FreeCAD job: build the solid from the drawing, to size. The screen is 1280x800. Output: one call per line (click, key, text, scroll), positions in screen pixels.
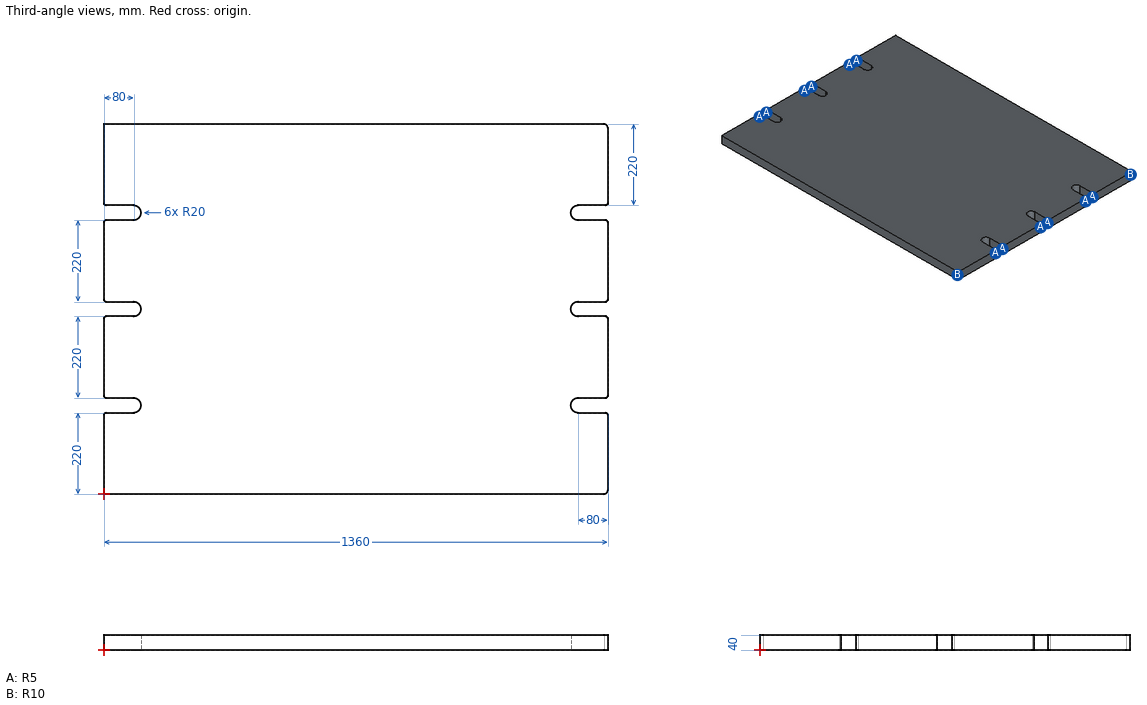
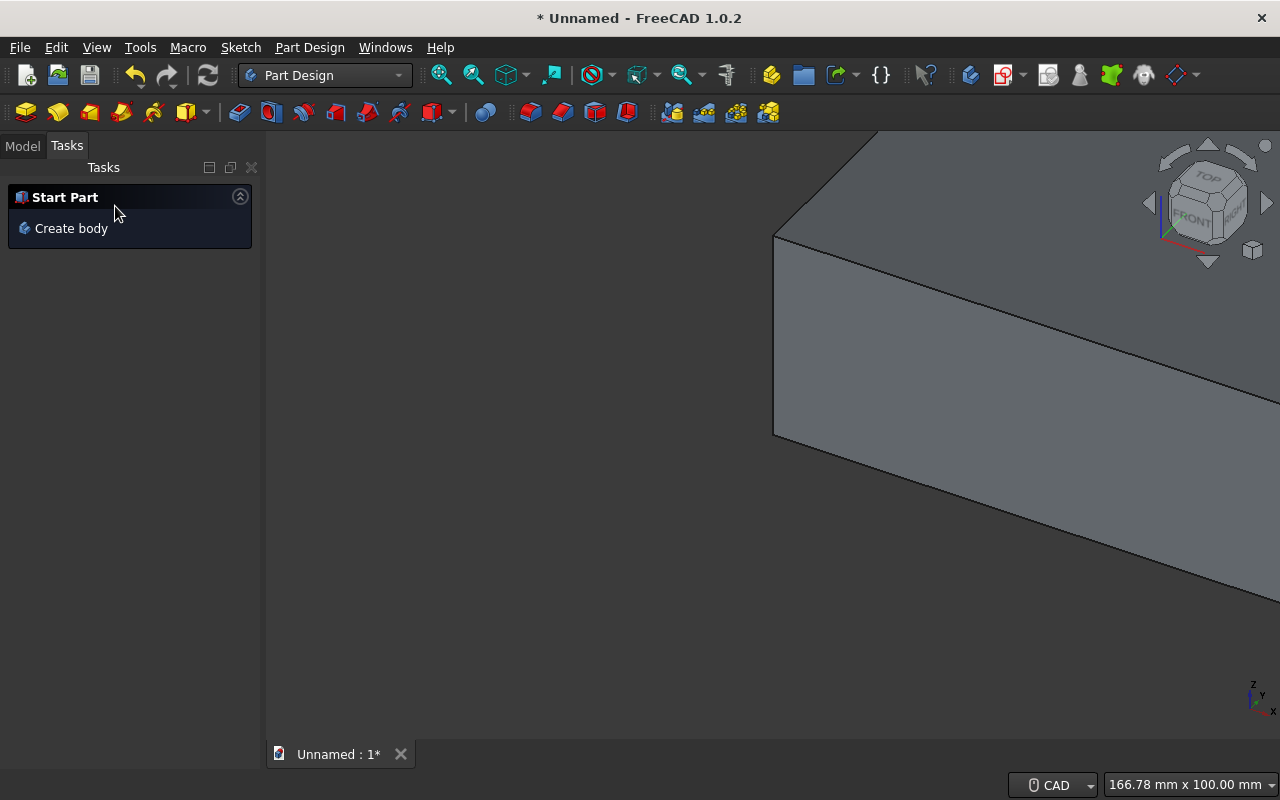
click(442, 76)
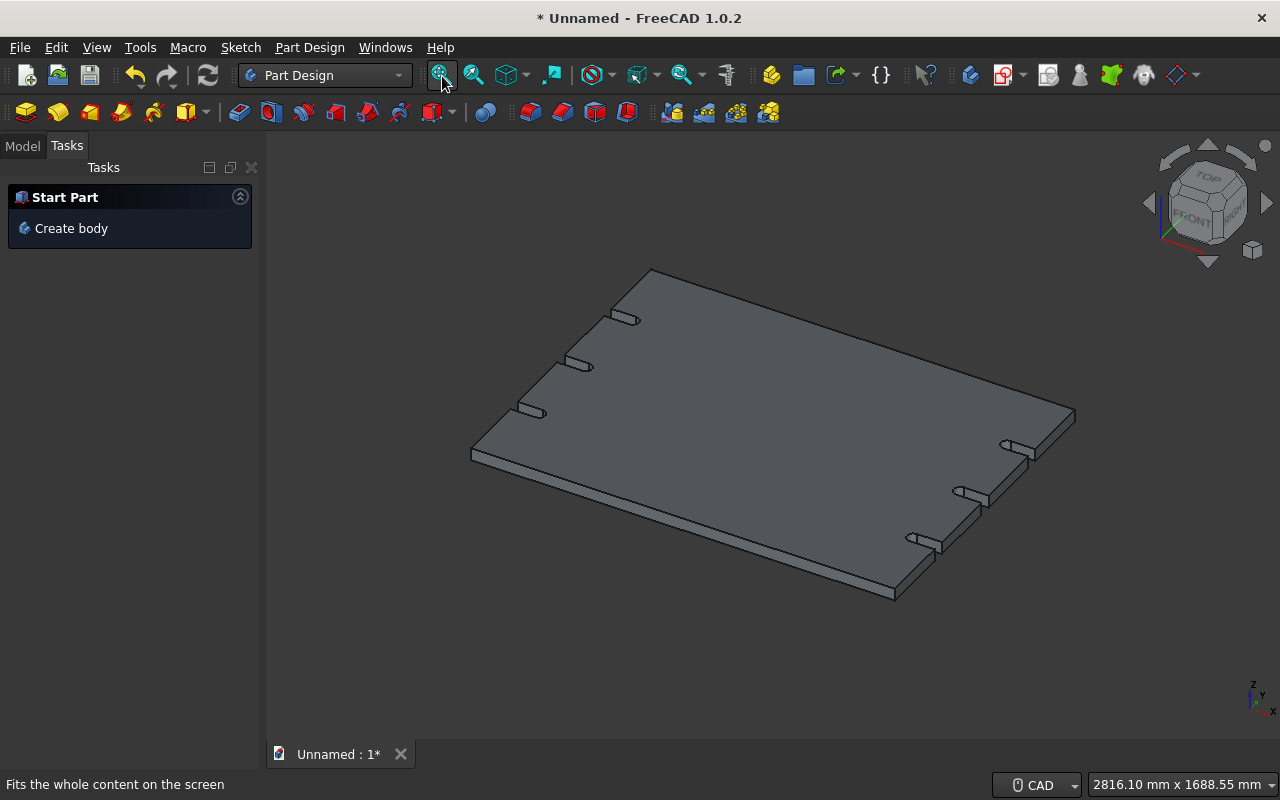
click(1035, 455)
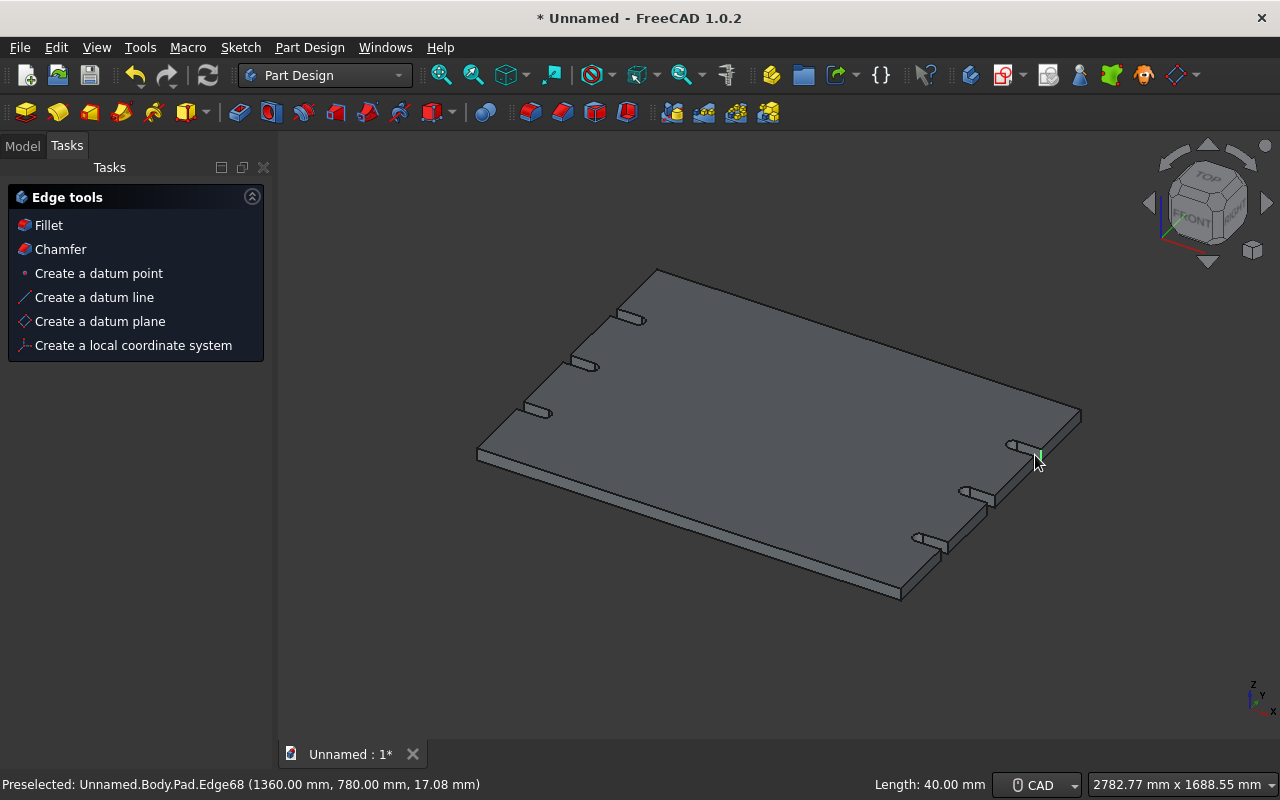
click(995, 501, ctrl)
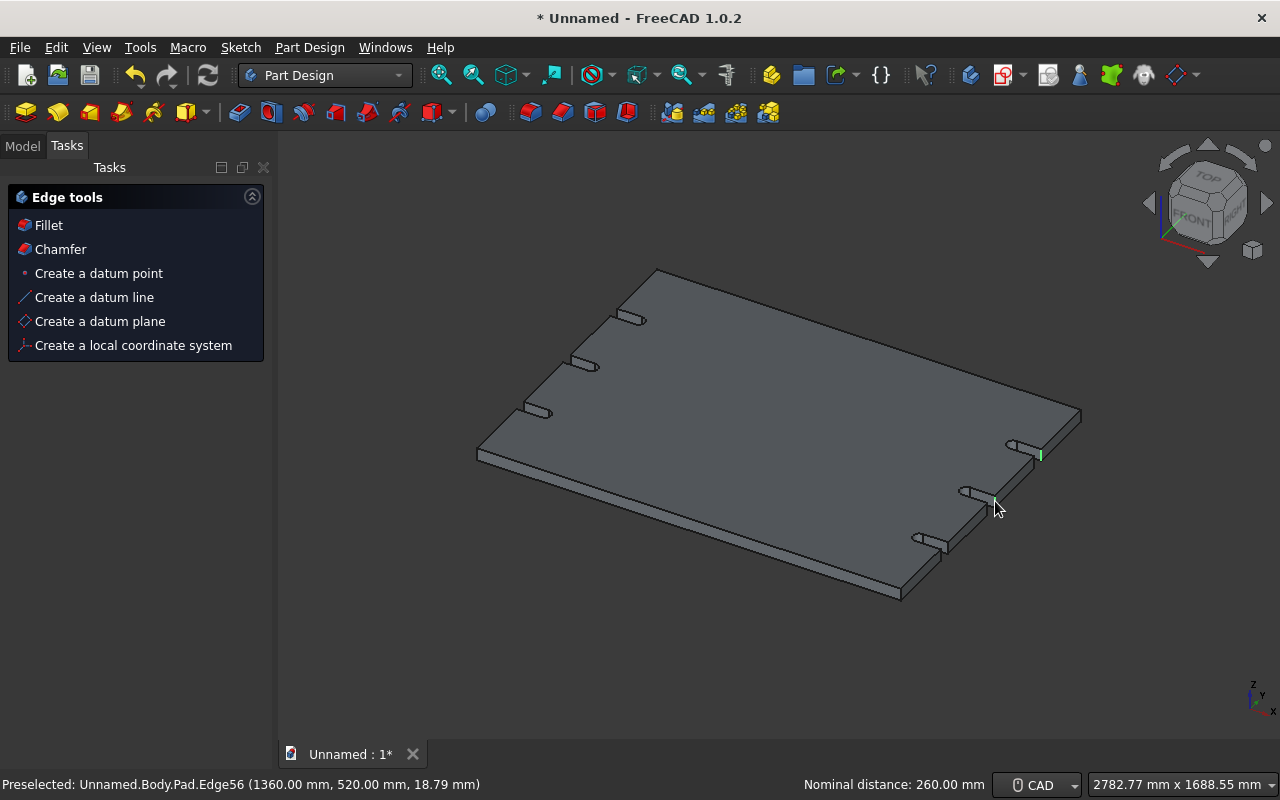
click(948, 548, ctrl)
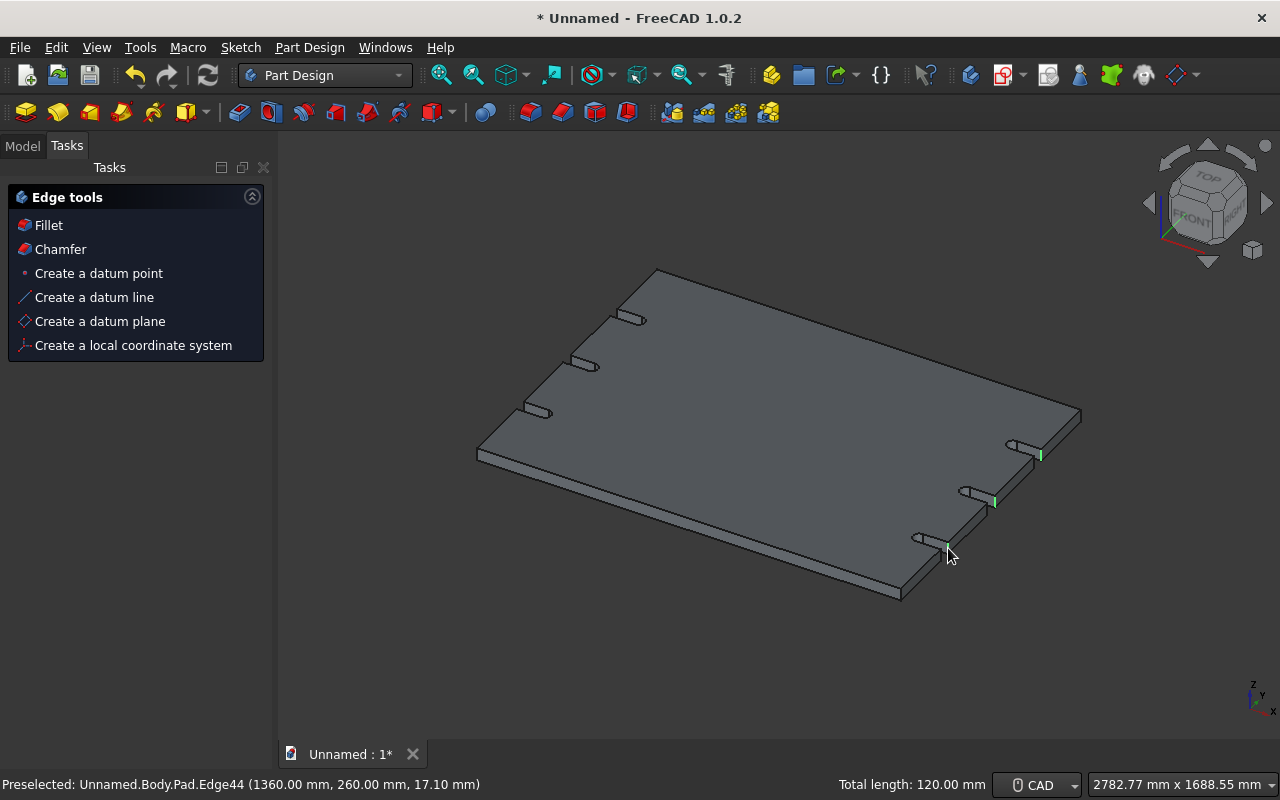
scroll(517, 414, up, 6)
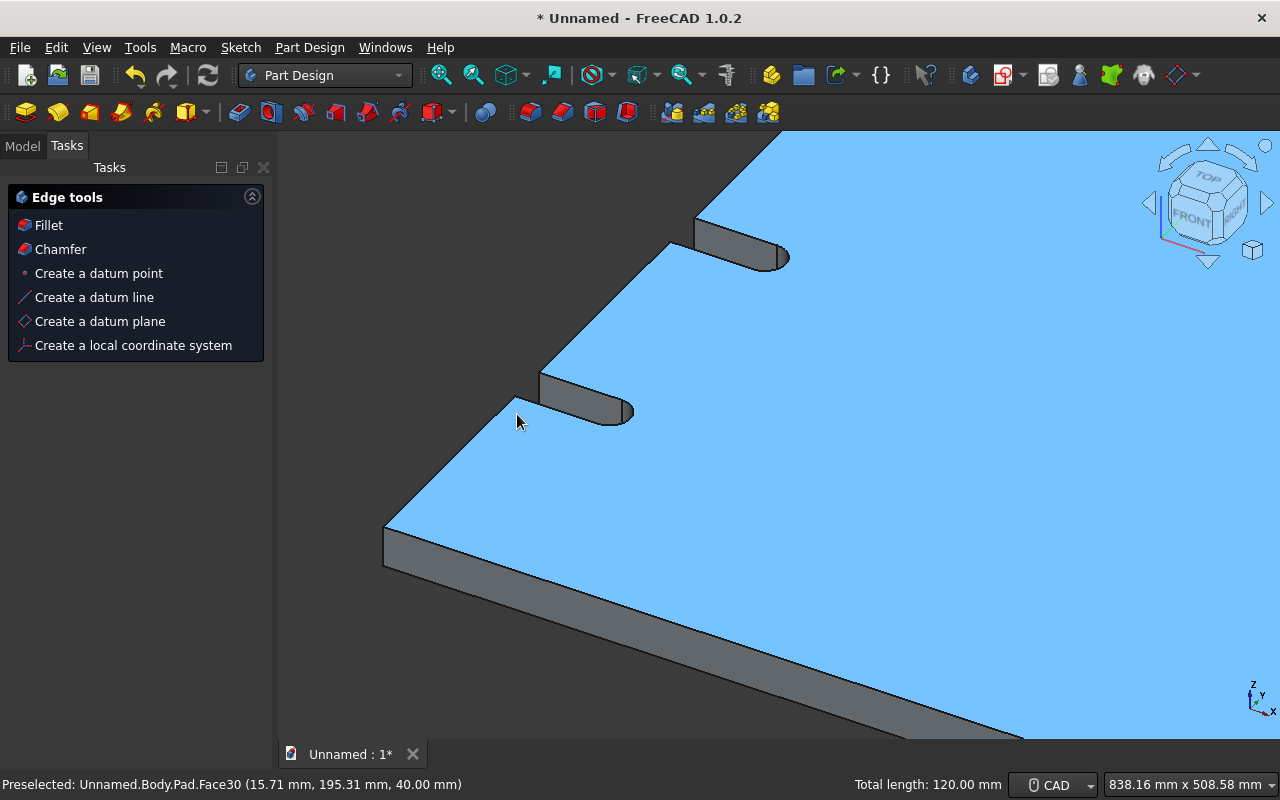
click(442, 76)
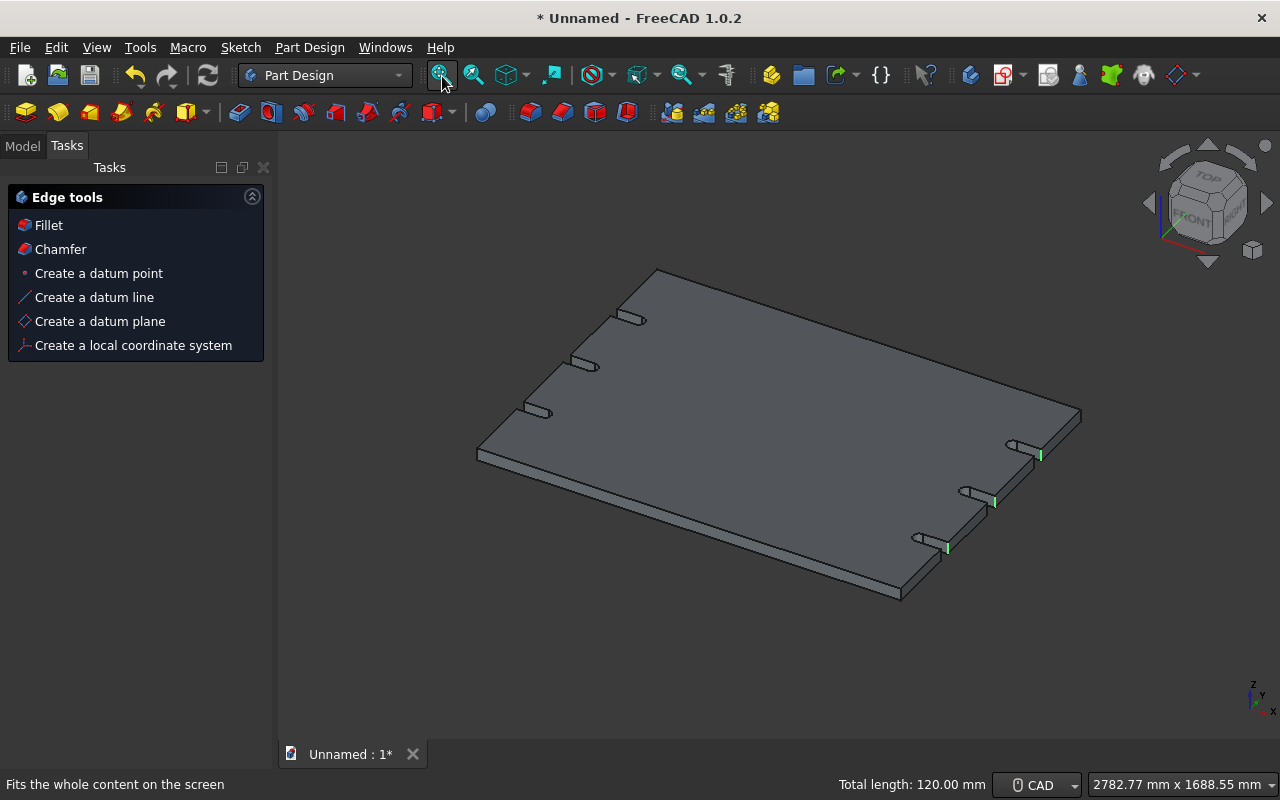
key(0)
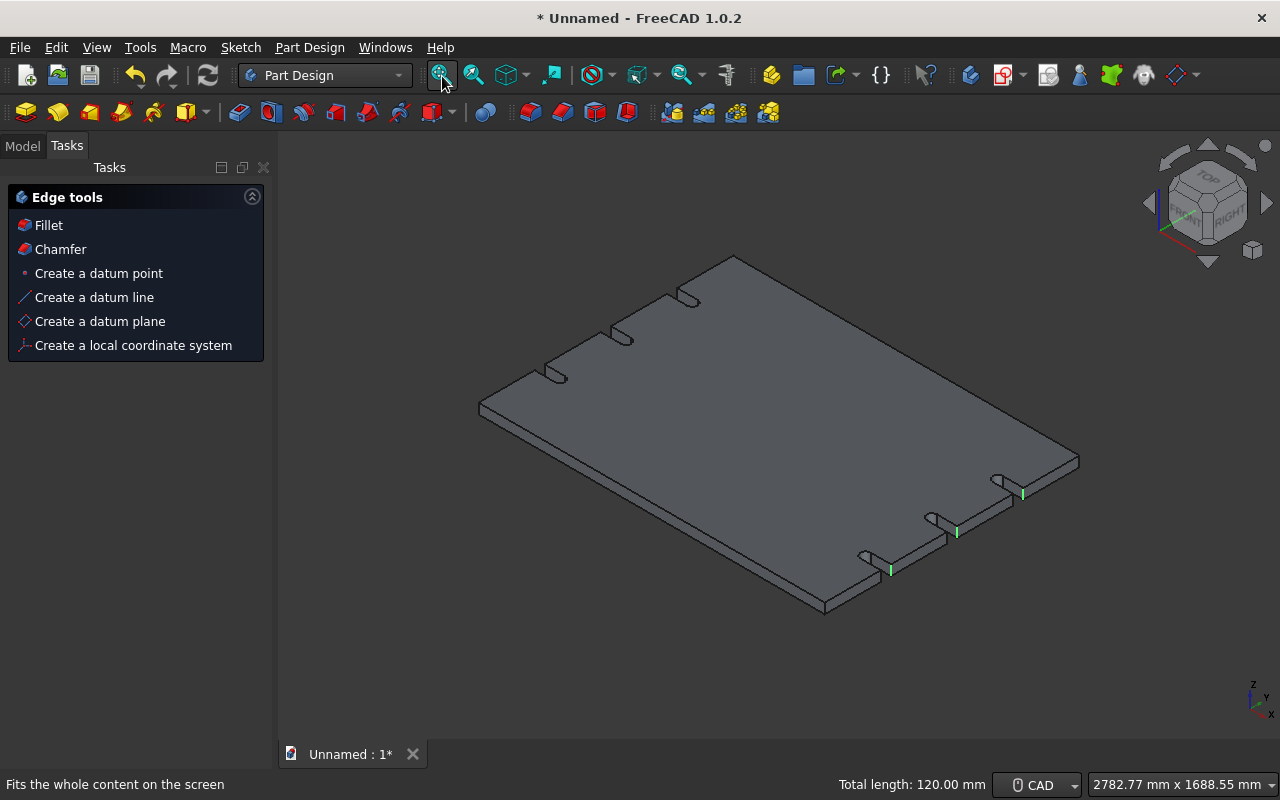
scroll(535, 375, up, 6)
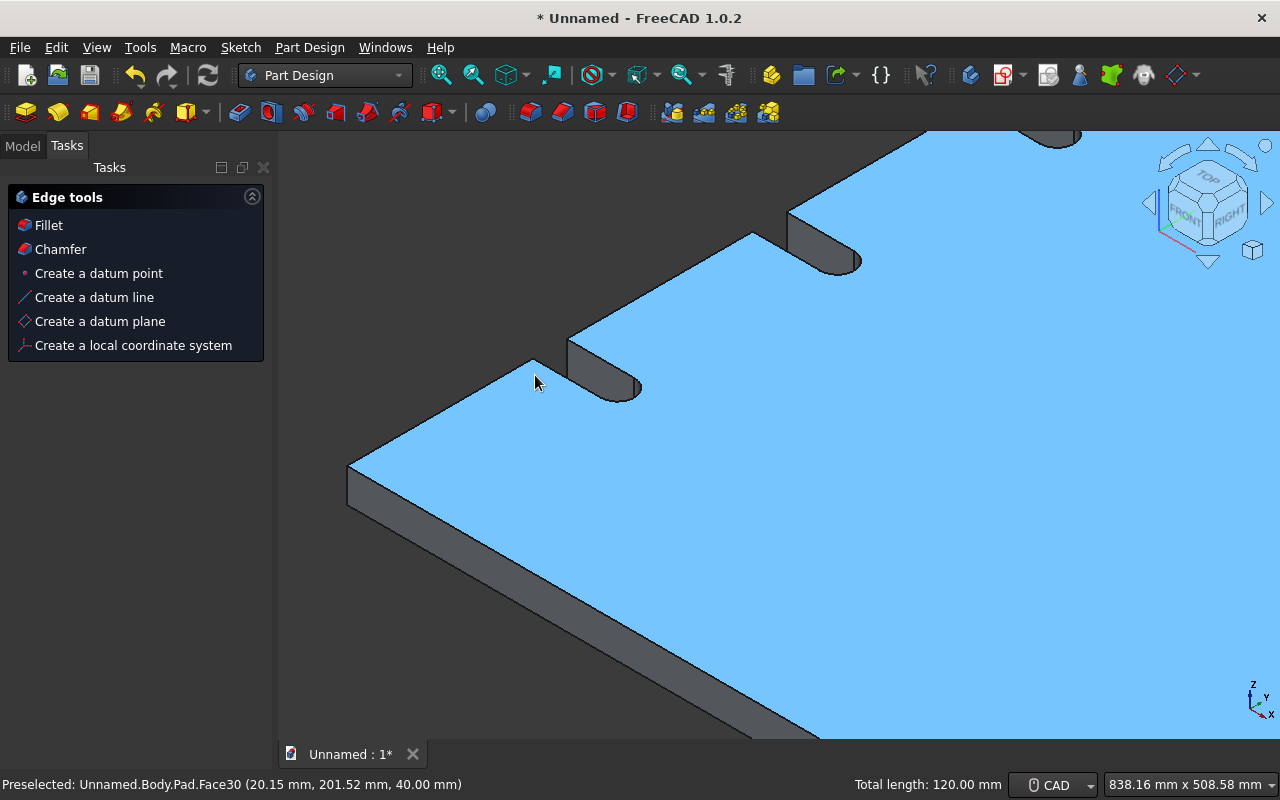
click(442, 76)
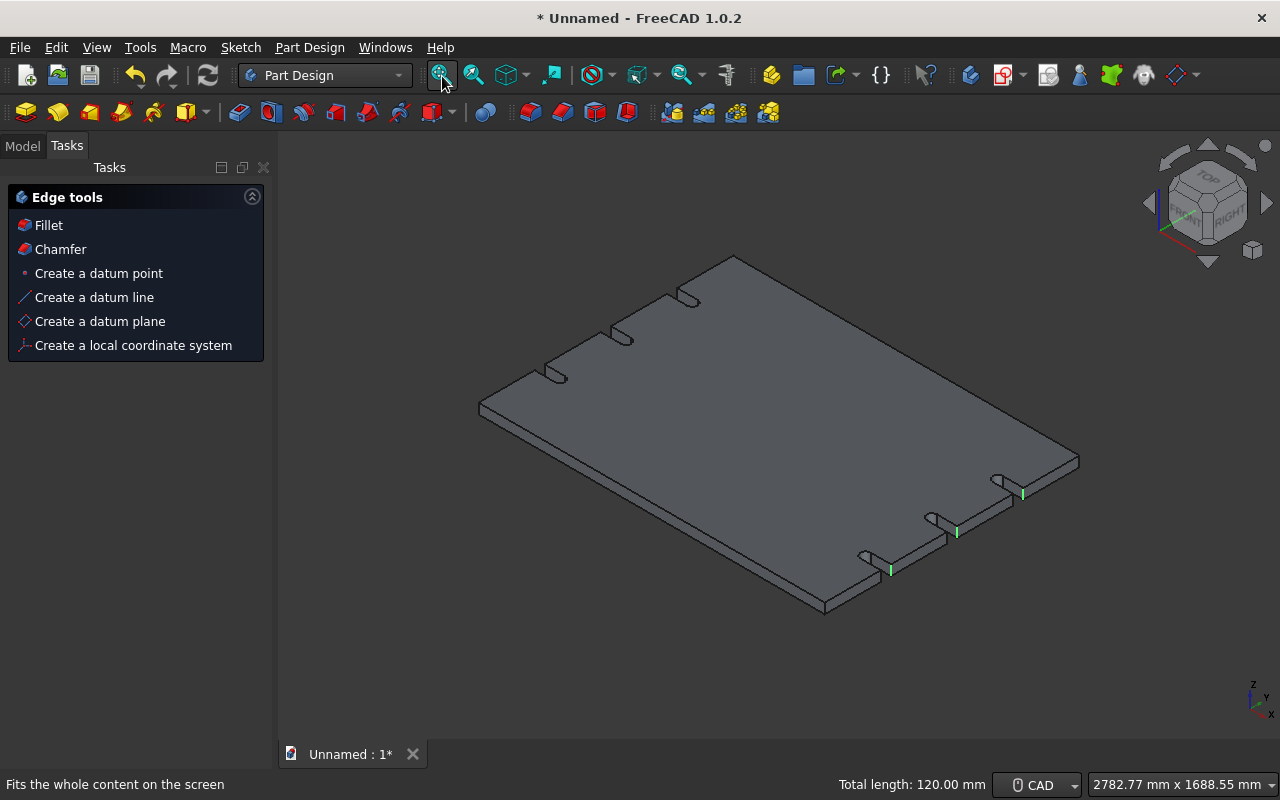
key(2)